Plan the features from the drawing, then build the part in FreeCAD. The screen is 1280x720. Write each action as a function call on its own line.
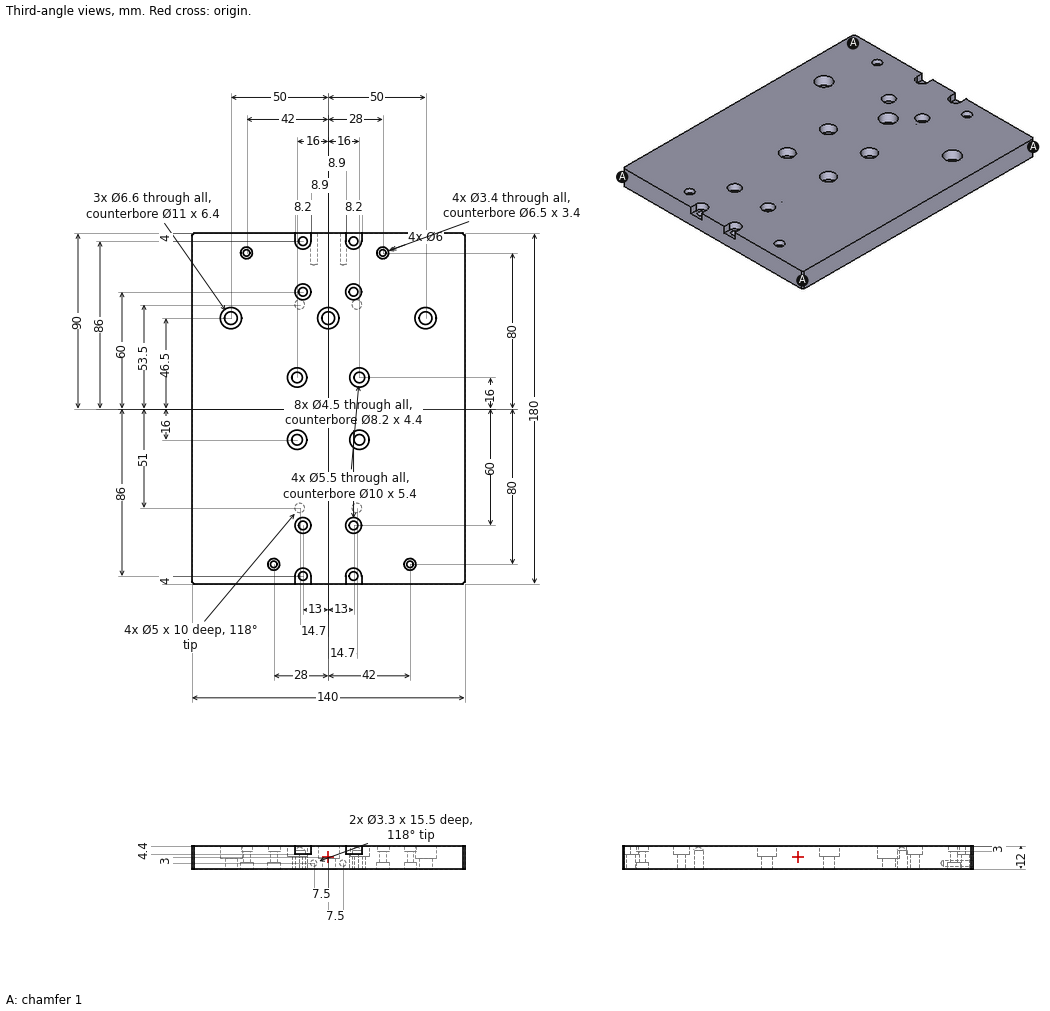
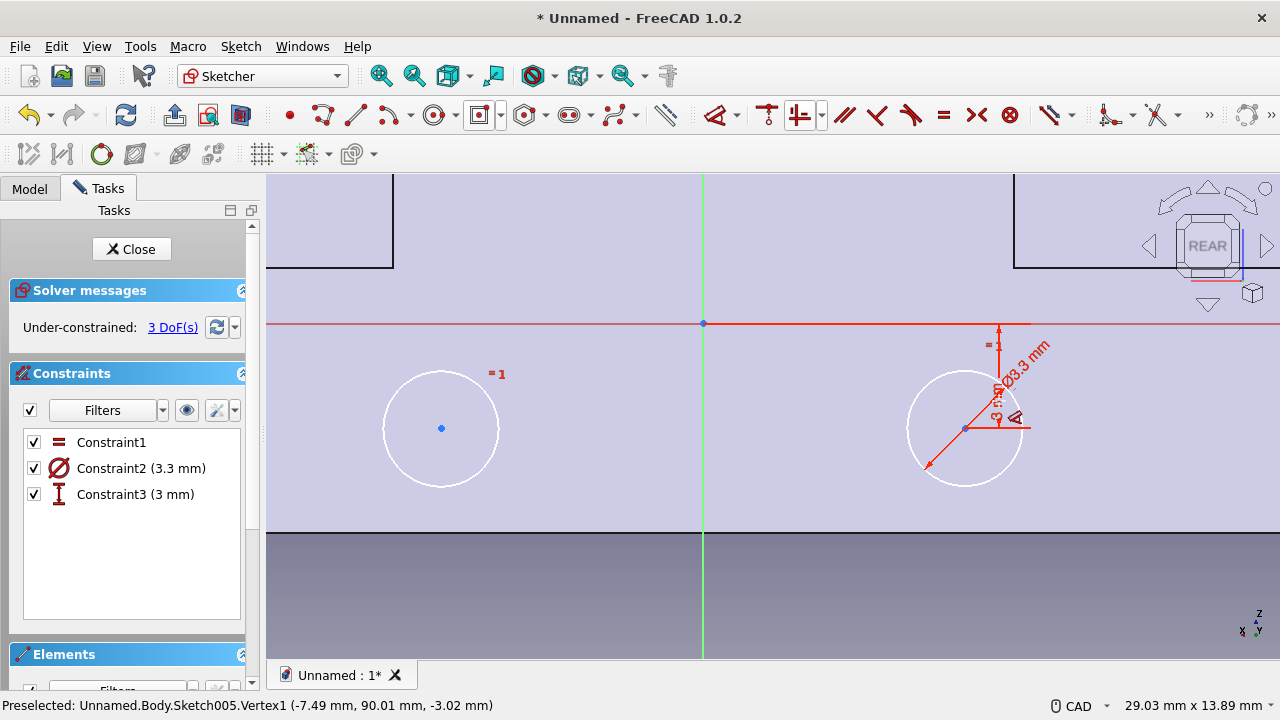
click(441, 429)
click(407, 352)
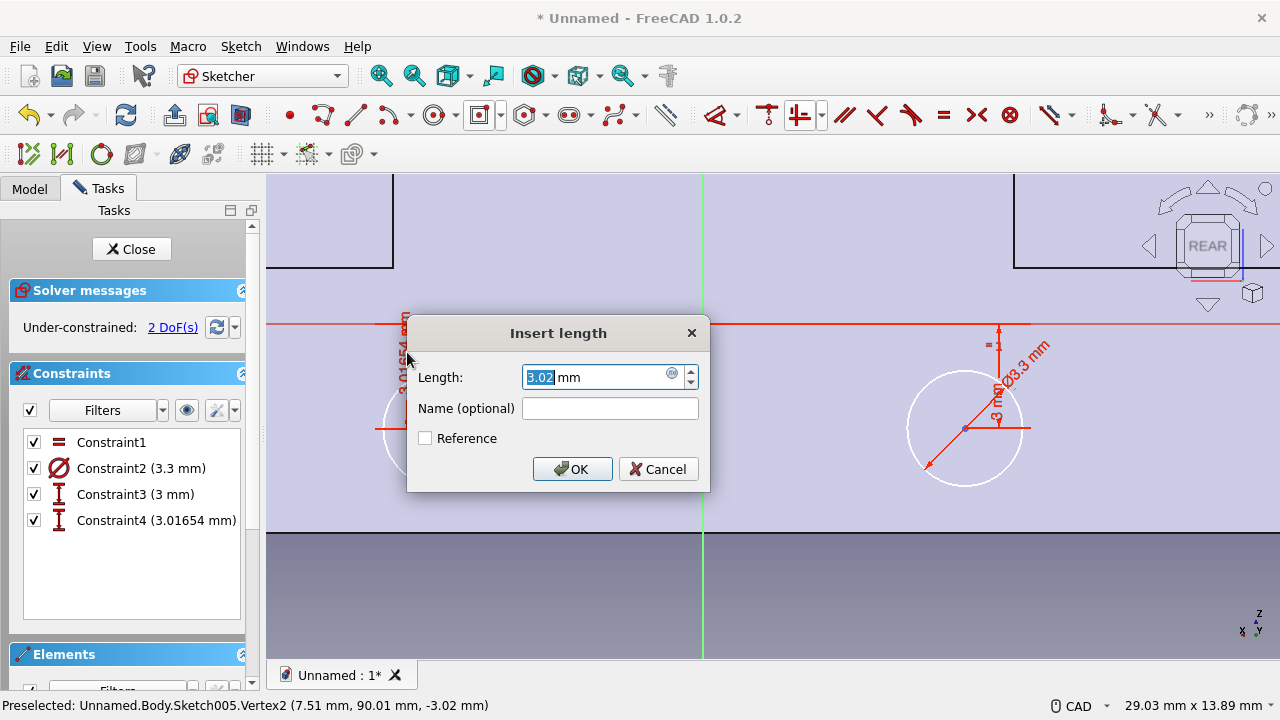
text(3)
key(Return)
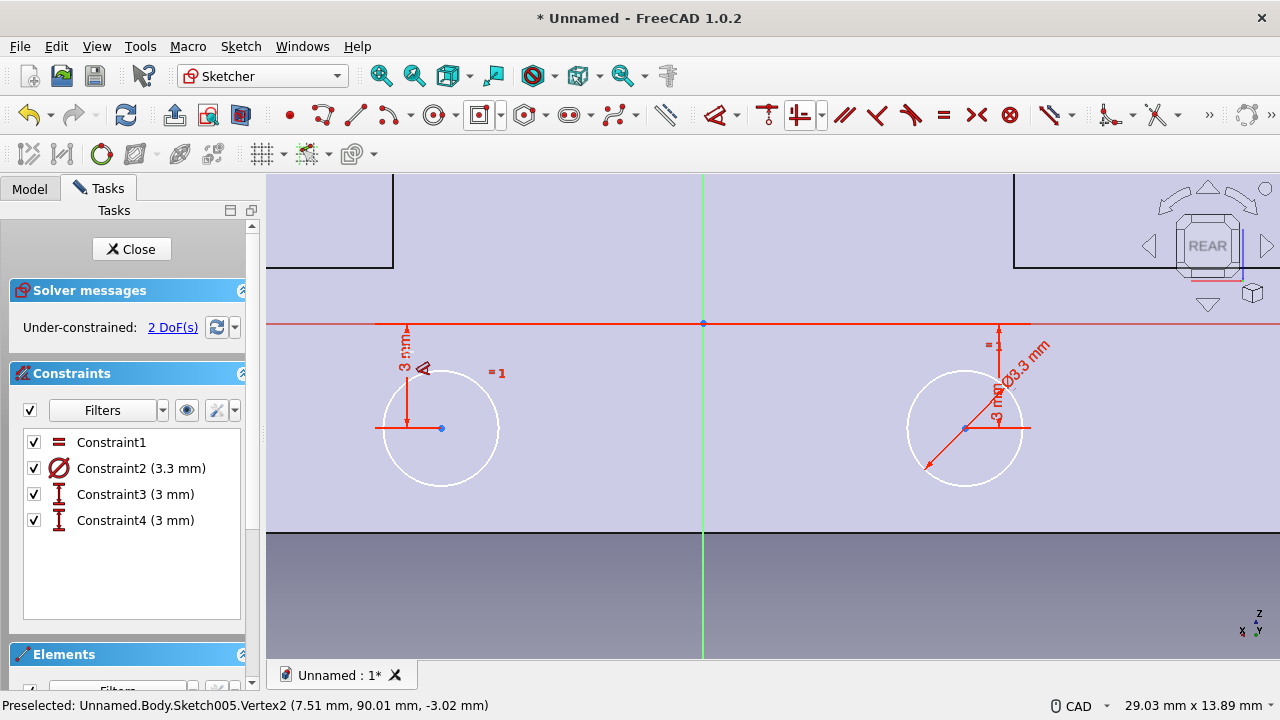
click(965, 428)
click(834, 290)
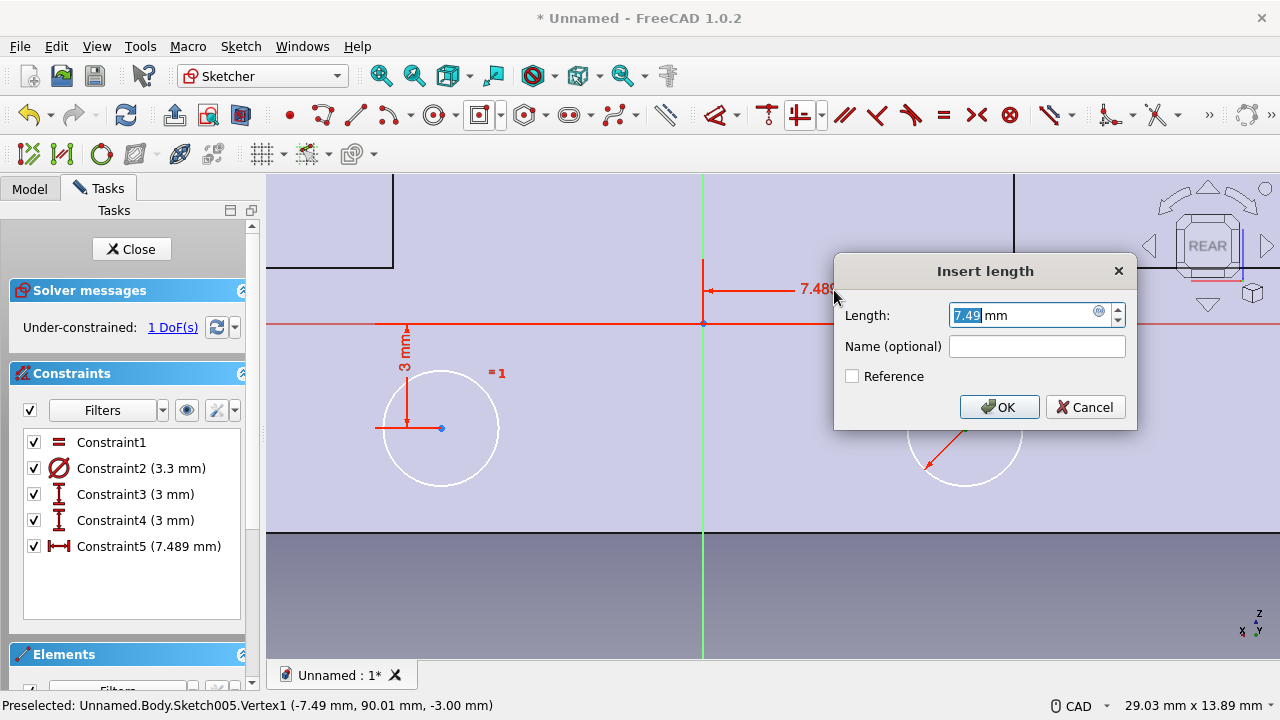
text(7.5)
key(Return)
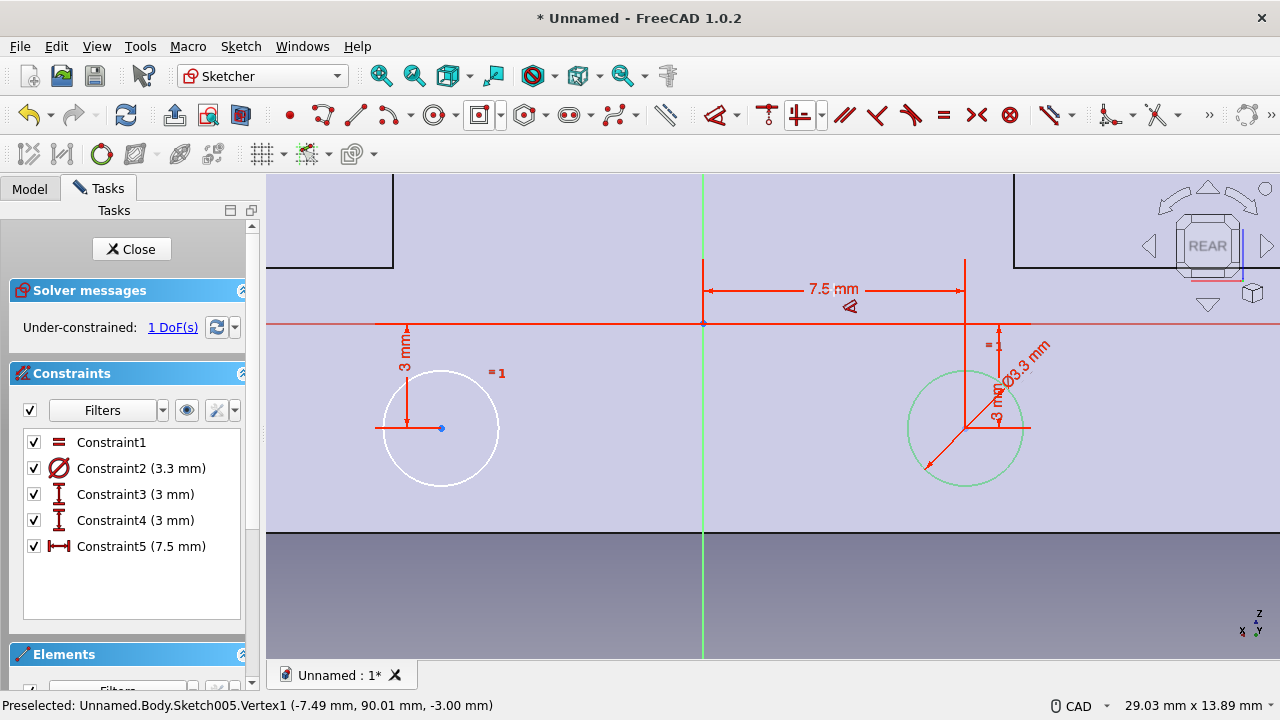
click(441, 428)
click(572, 290)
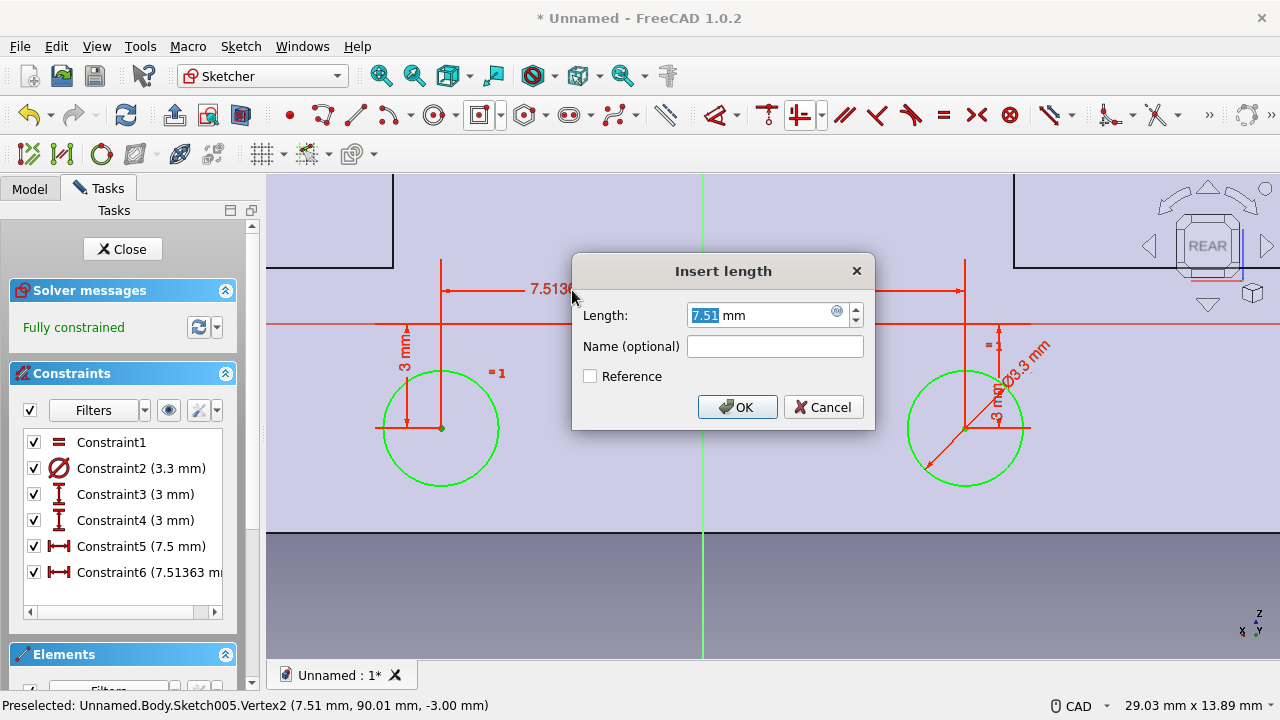
text(7.5)
key(Return)
key(Escape)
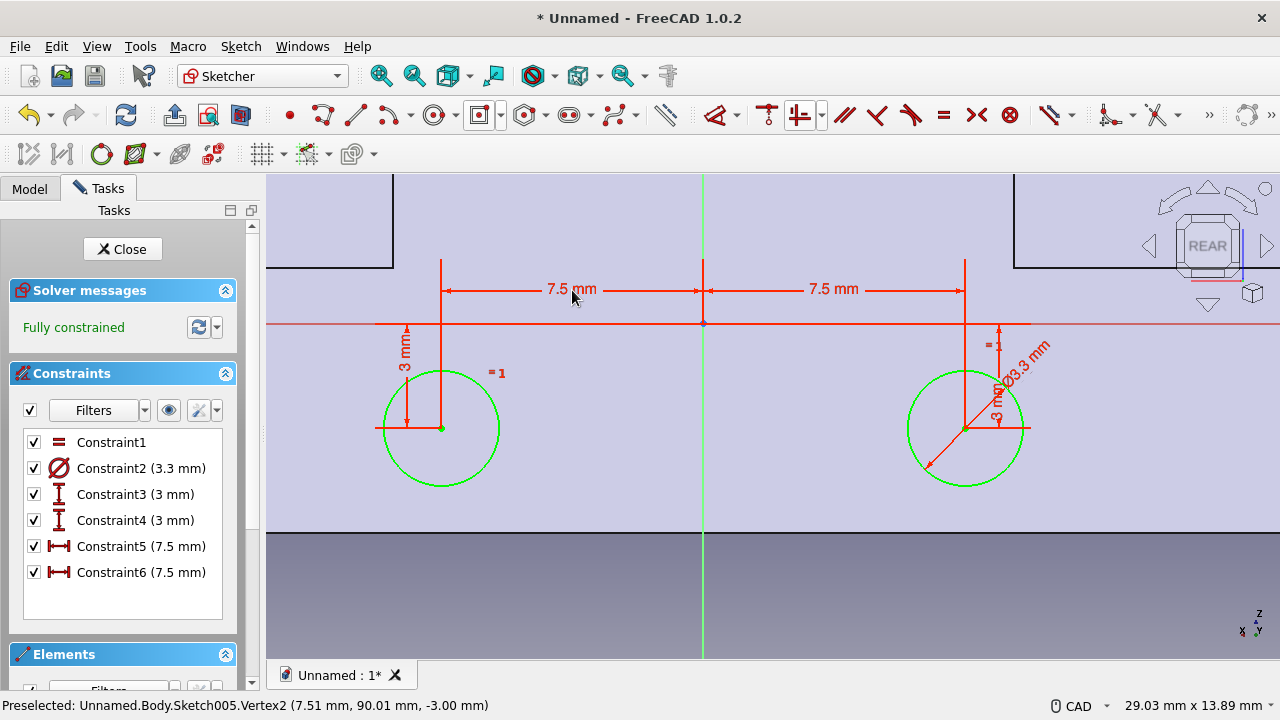
click(123, 249)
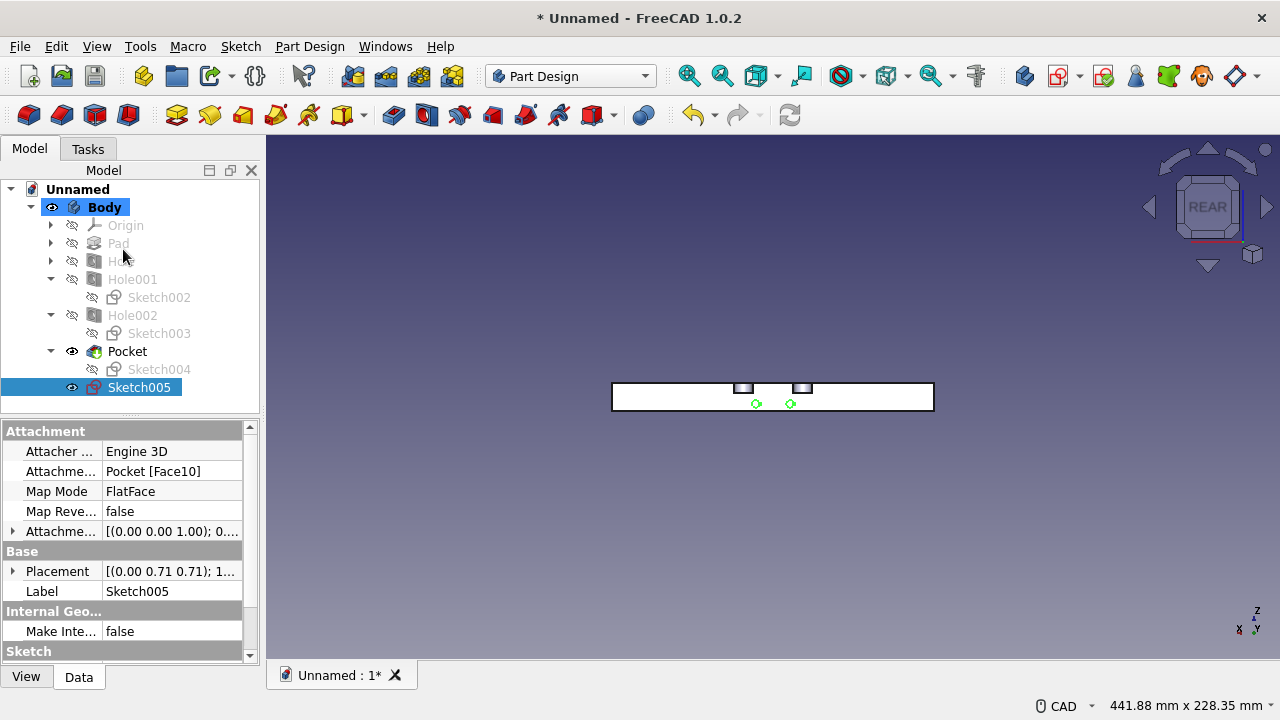
click(427, 116)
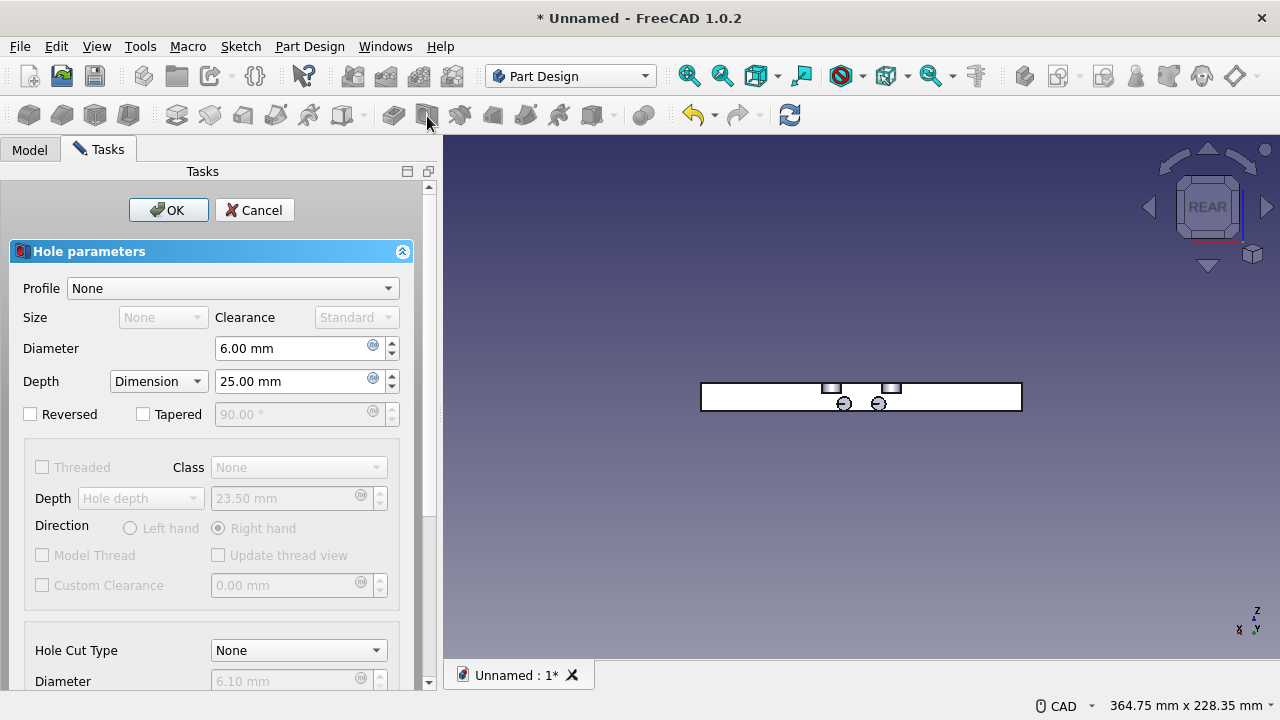
triple_click(300, 348)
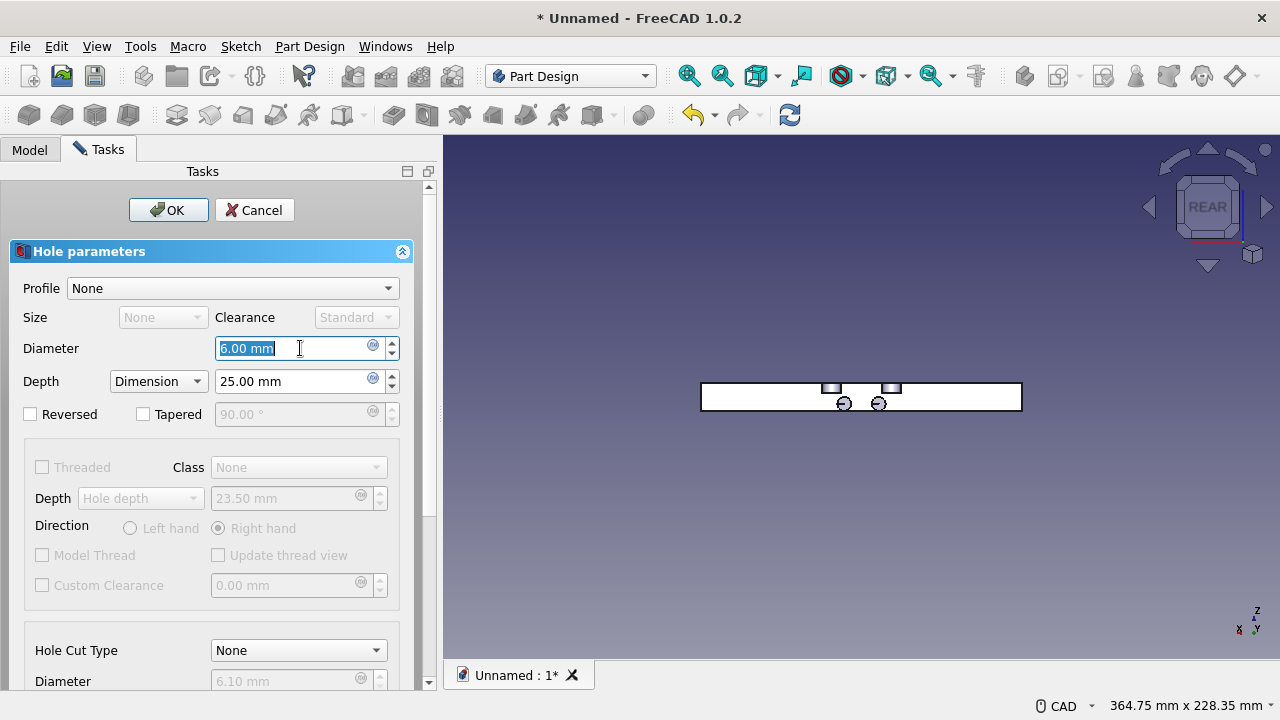
text(3.3)
key(Tab)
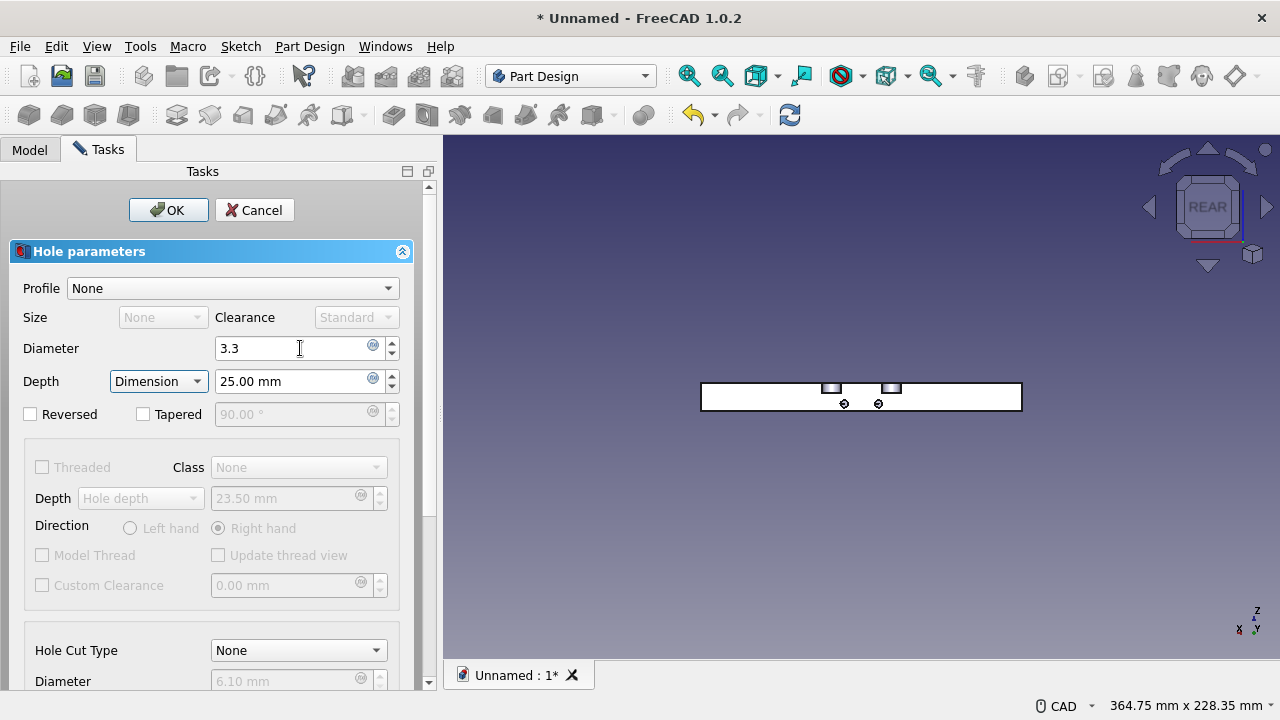
triple_click(300, 382)